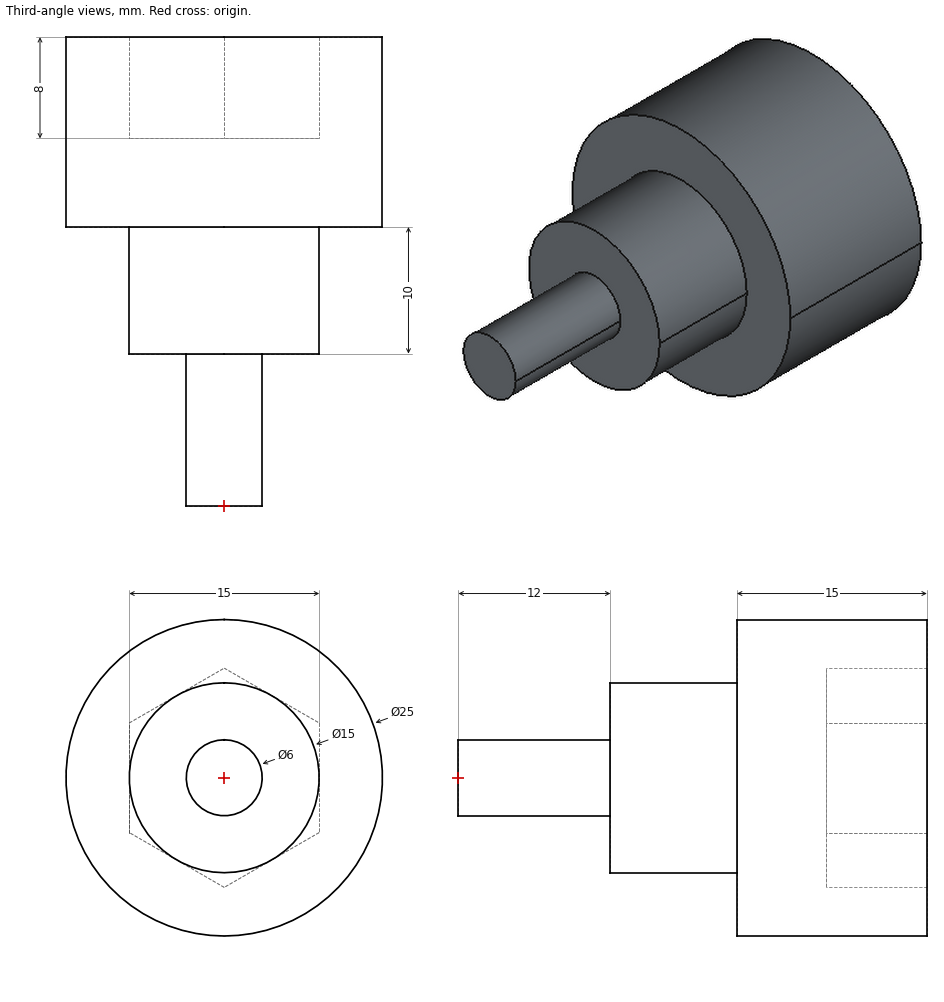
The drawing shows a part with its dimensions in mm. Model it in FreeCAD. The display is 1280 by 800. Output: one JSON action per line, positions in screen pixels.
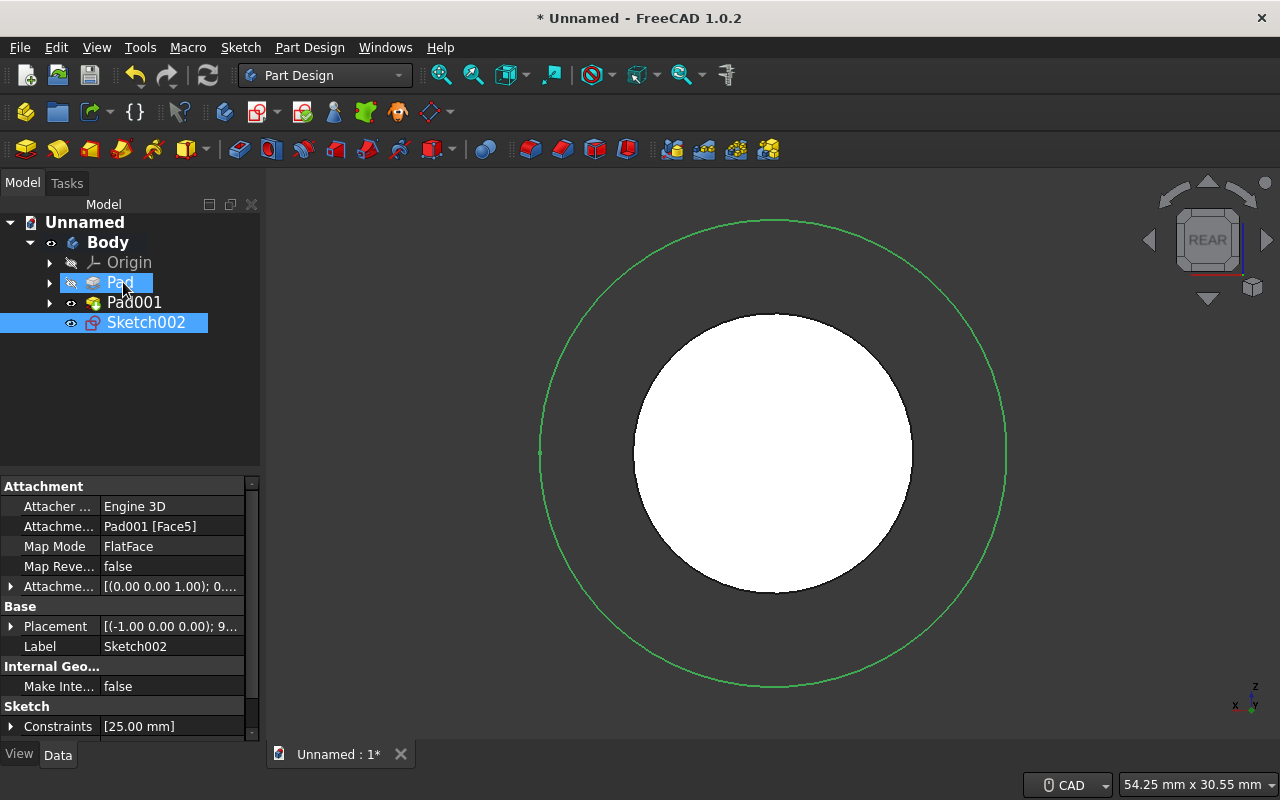
{"action": "left_click", "coordinate": [26, 150]}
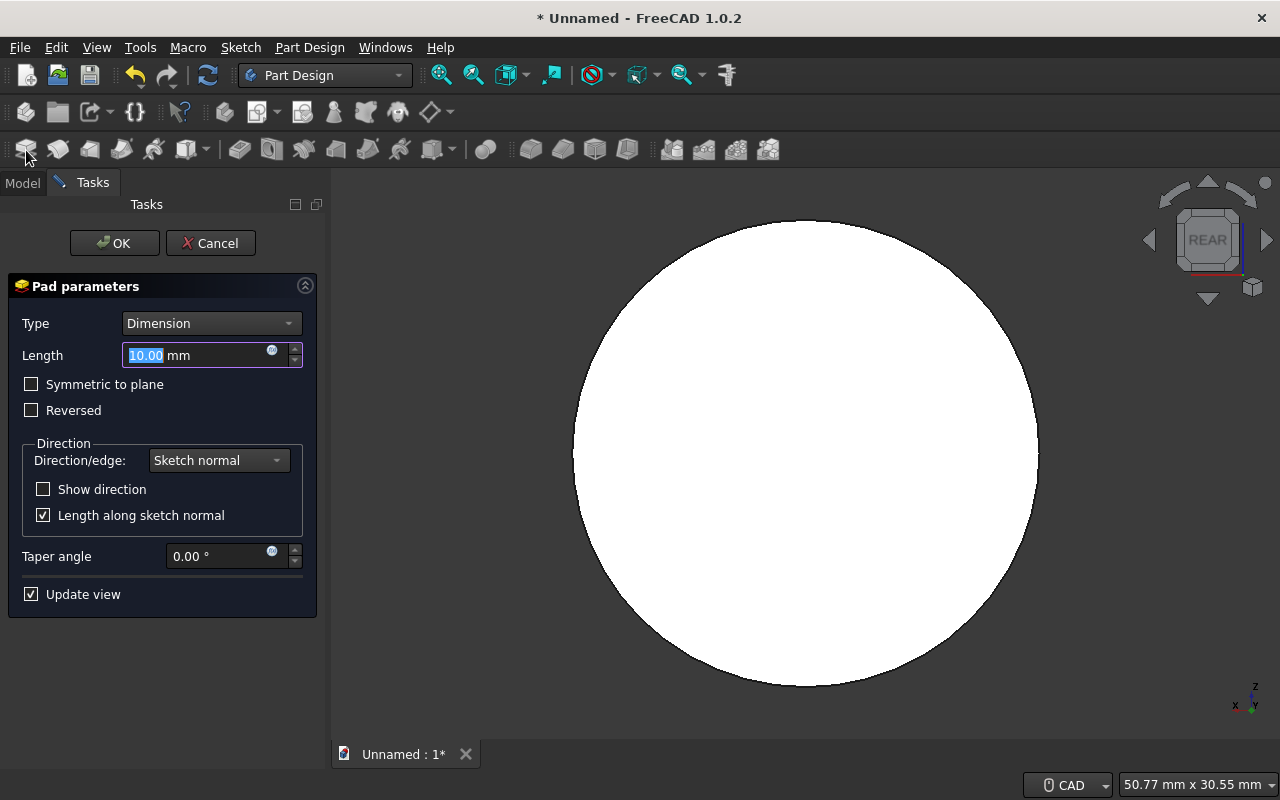
{"action": "type", "text": "15"}
{"action": "key", "text": "Tab"}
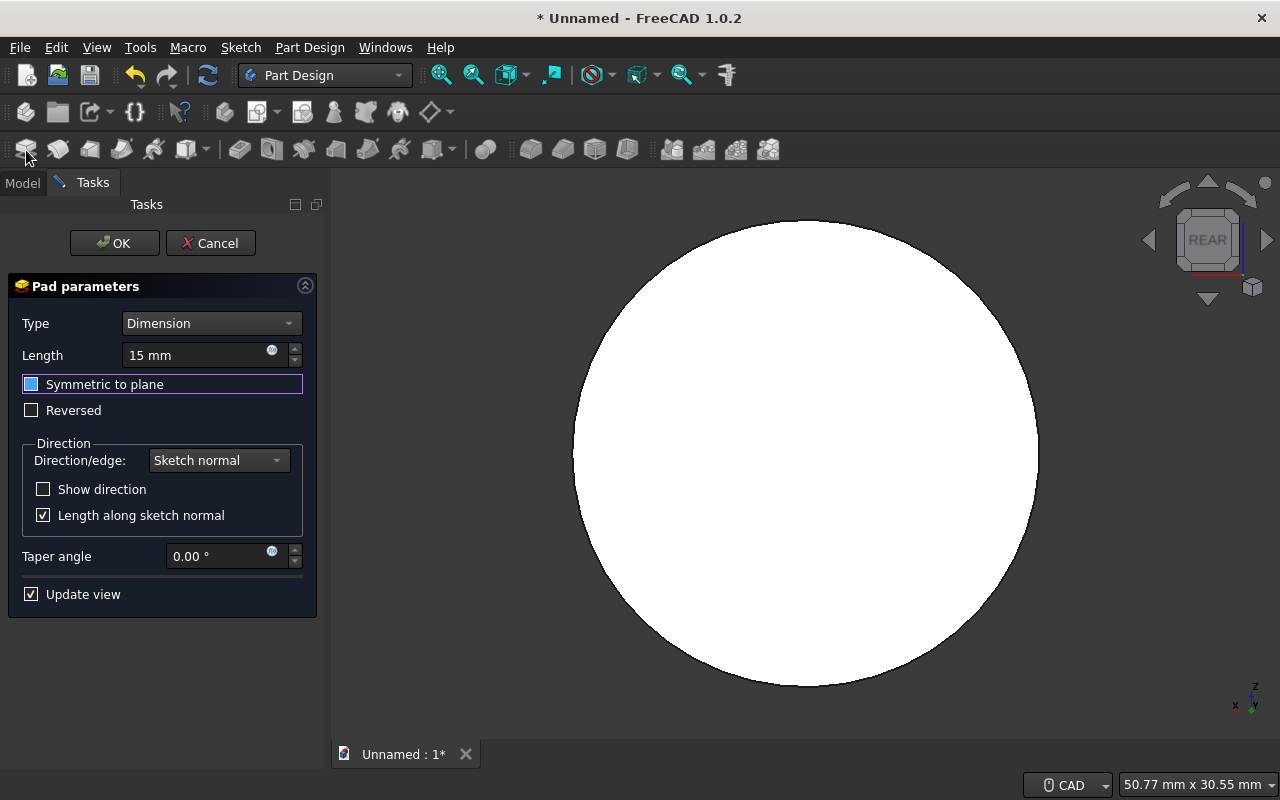
{"action": "left_click", "coordinate": [115, 243]}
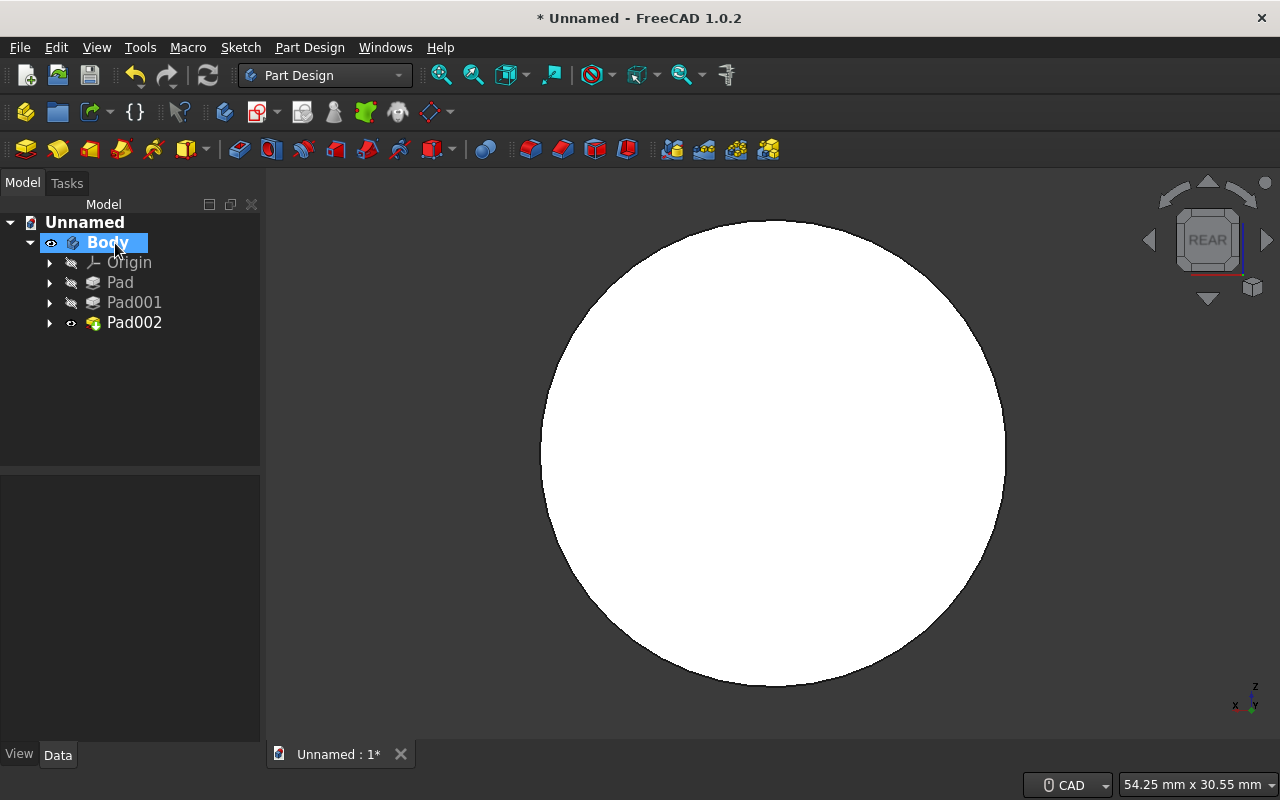
{"action": "left_click", "coordinate": [773, 452]}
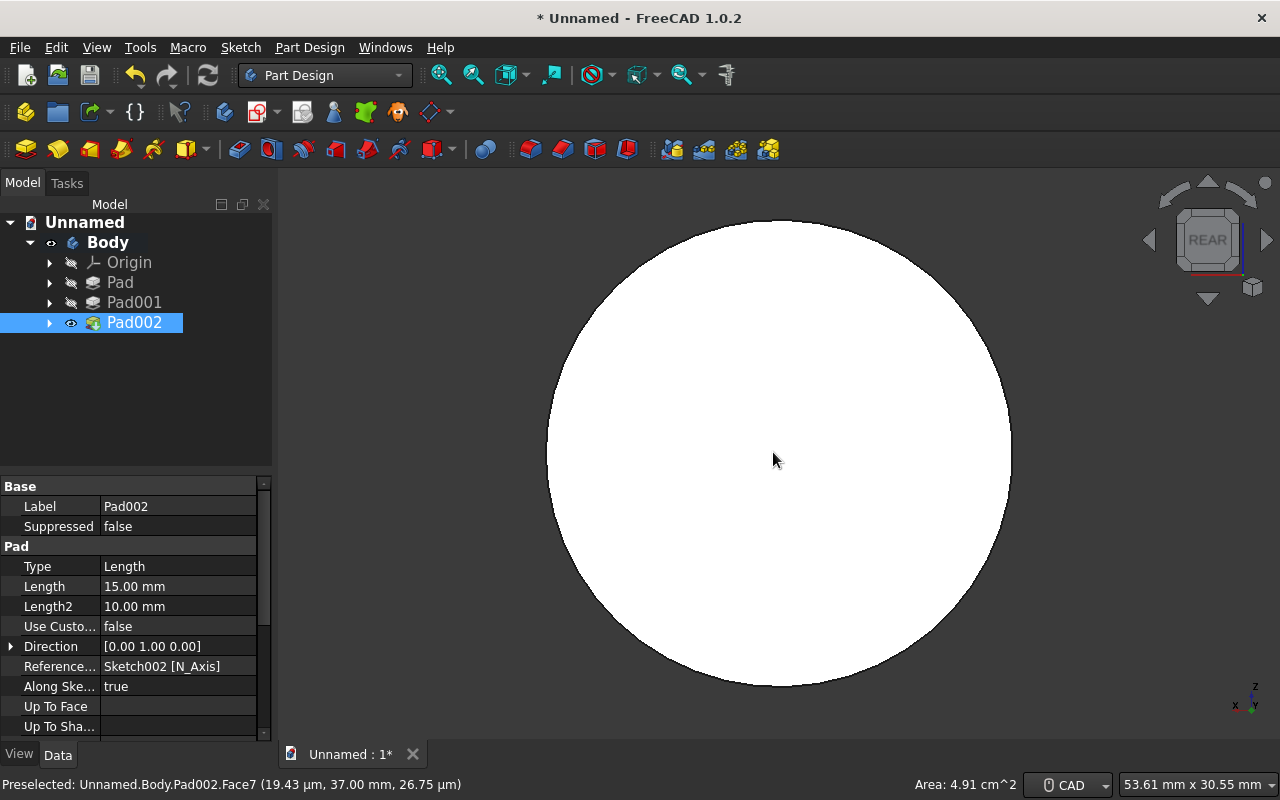
{"action": "left_click", "coordinate": [258, 112]}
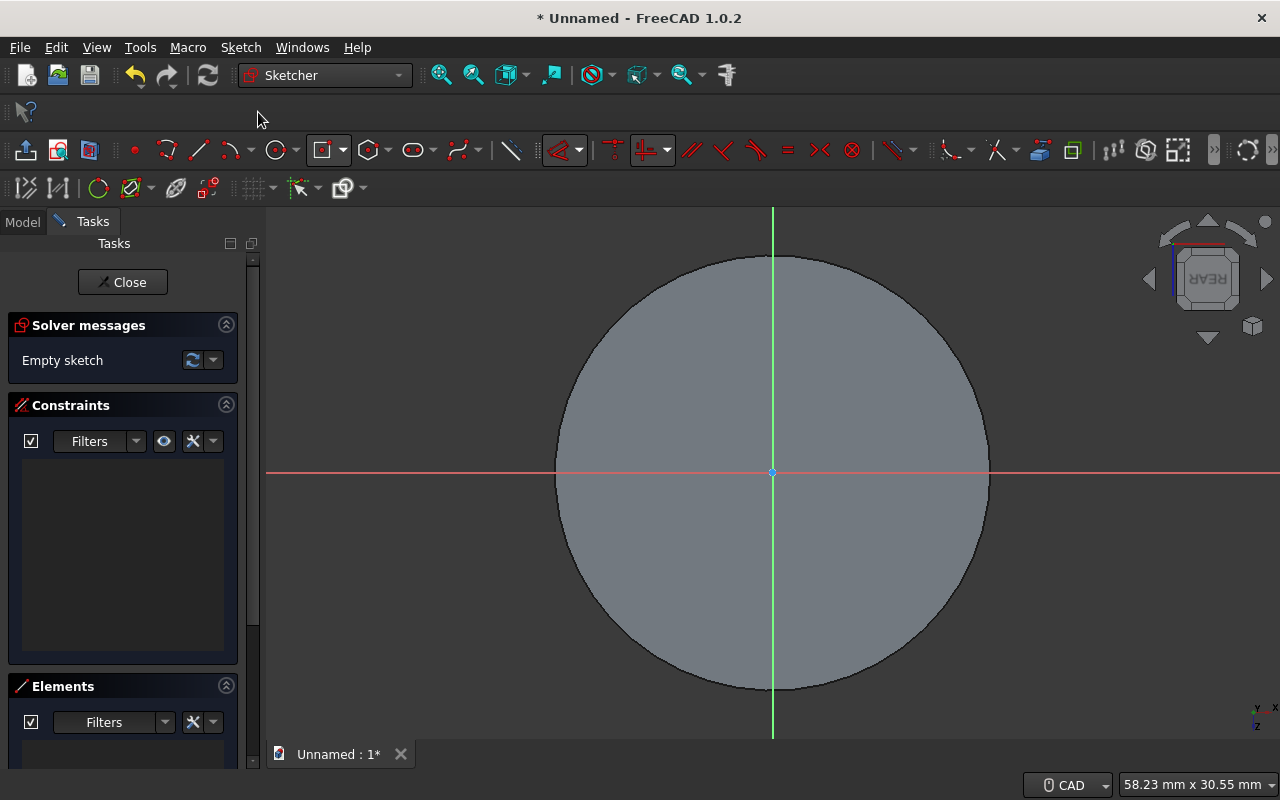
{"action": "left_click", "coordinate": [368, 150]}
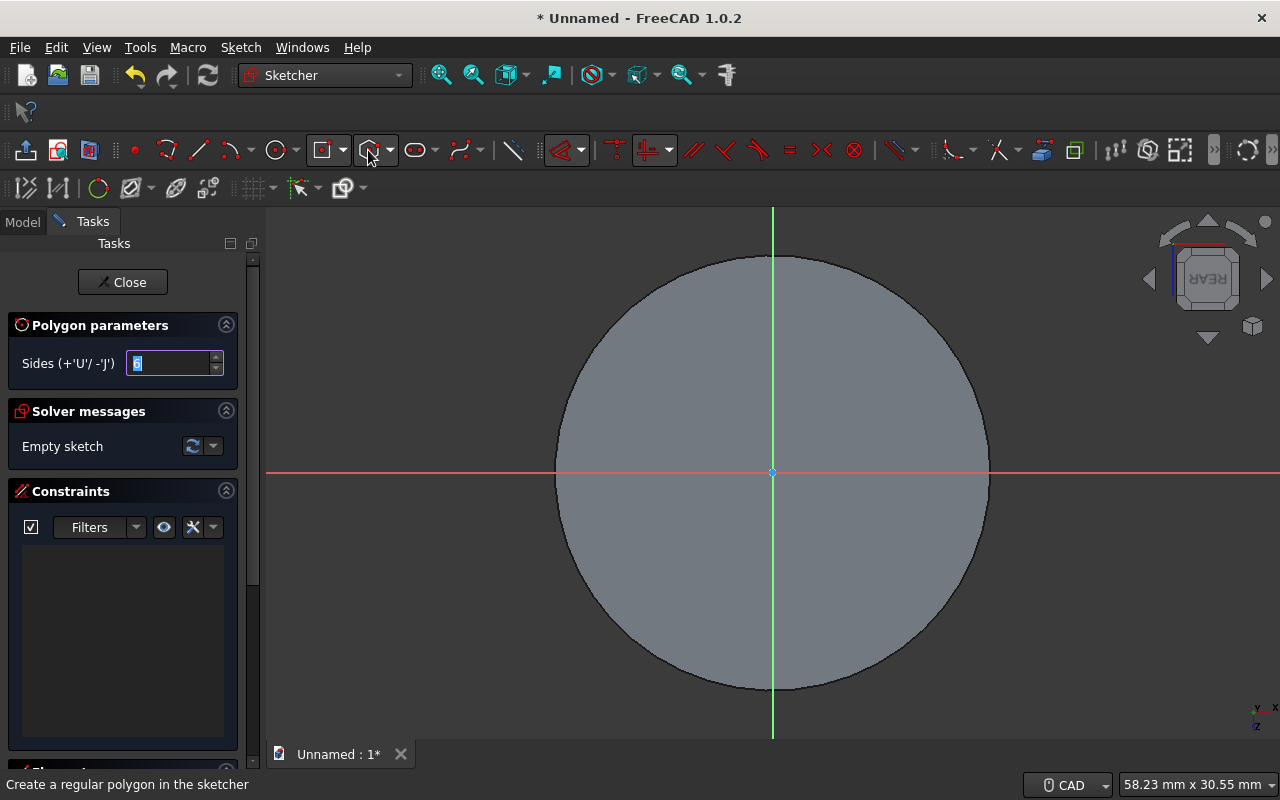
{"action": "left_click", "coordinate": [773, 473]}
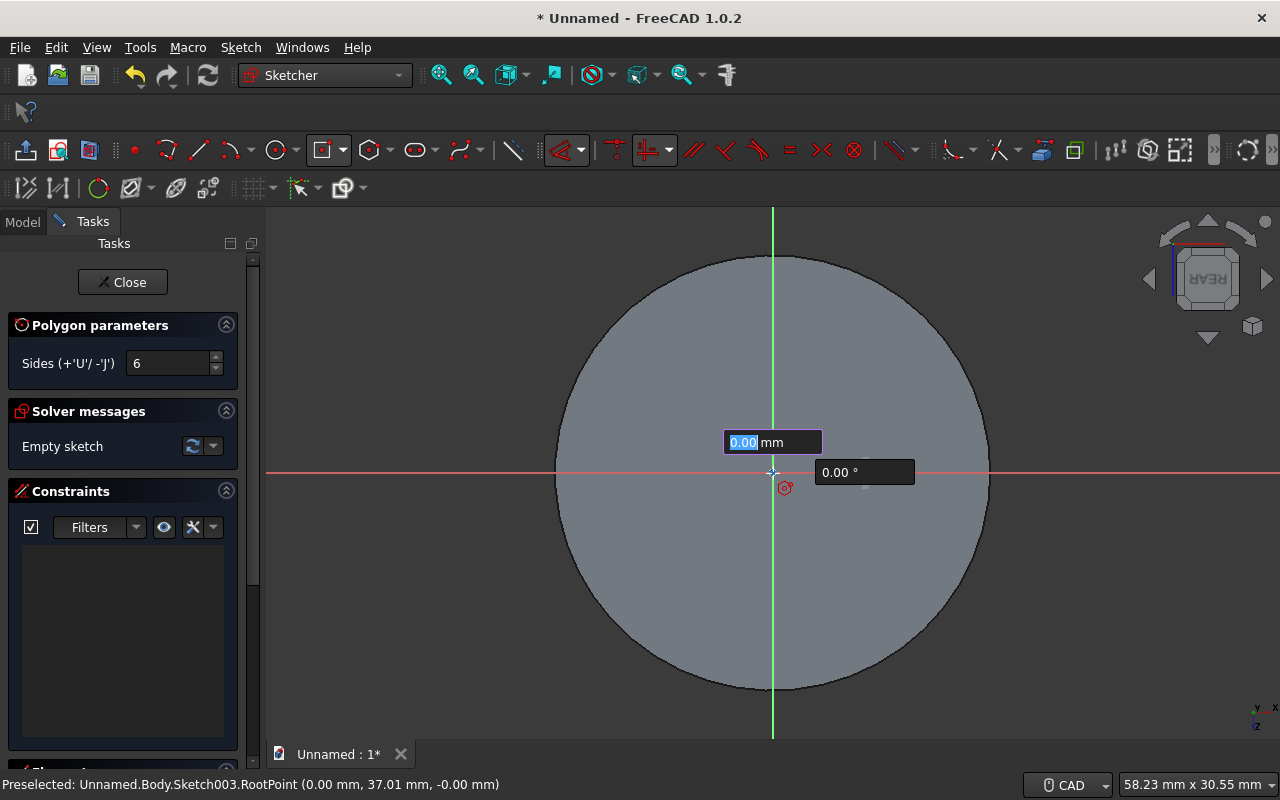
{"action": "left_click", "coordinate": [773, 322]}
{"action": "right_click", "coordinate": [773, 322]}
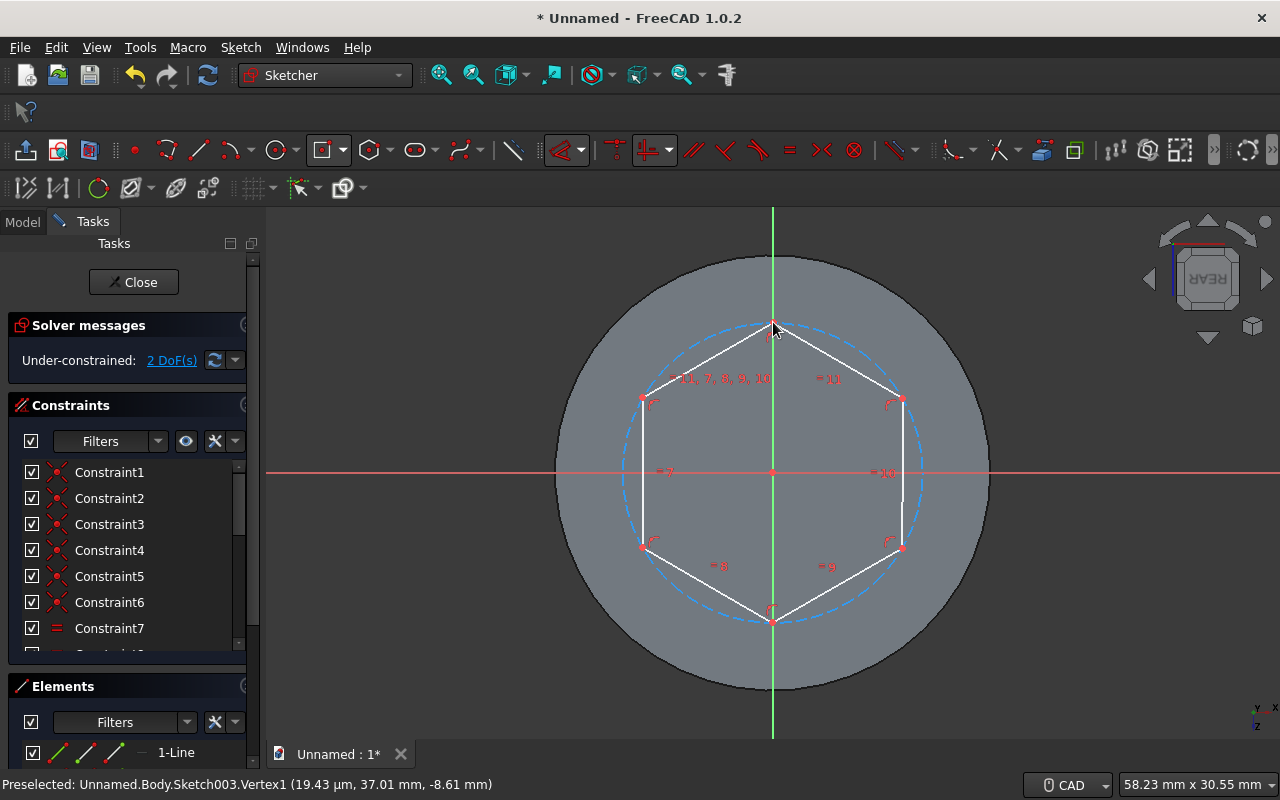
{"action": "left_click", "coordinate": [643, 443]}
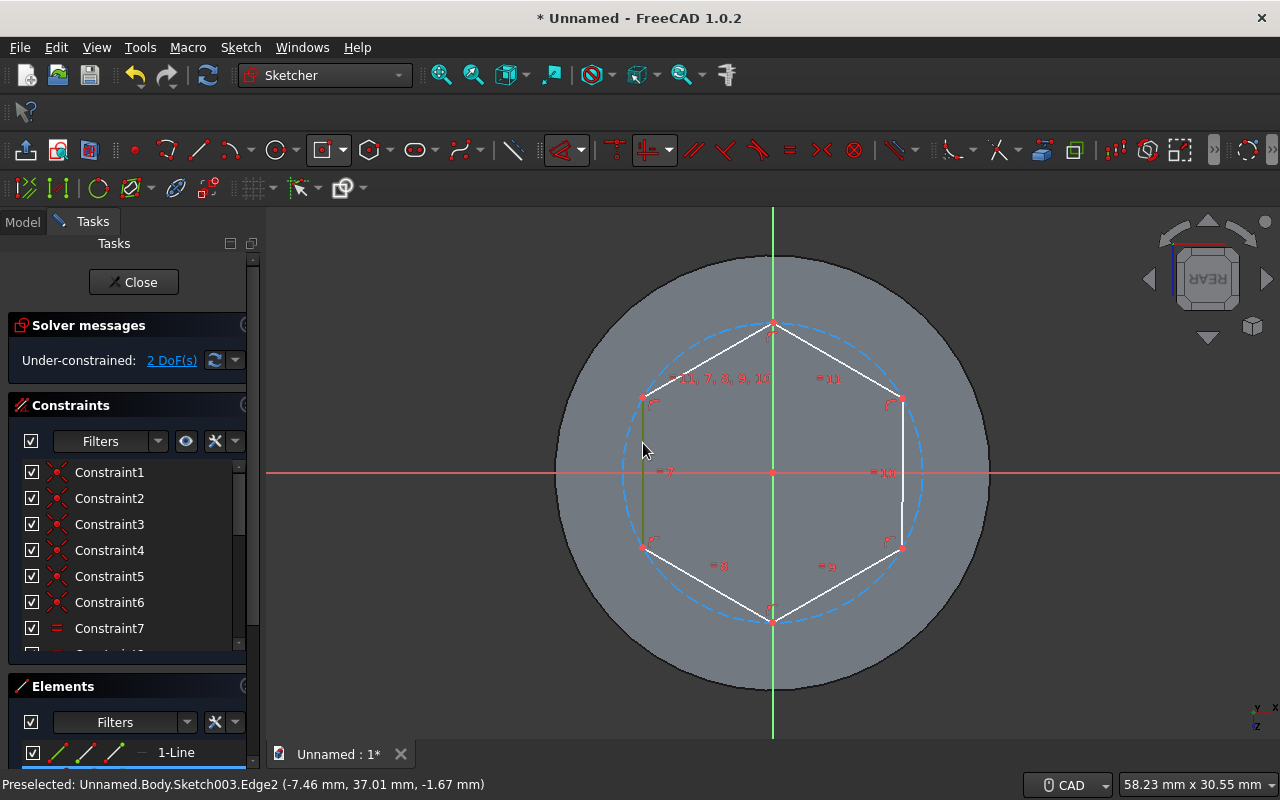
{"action": "key", "text": "v"}